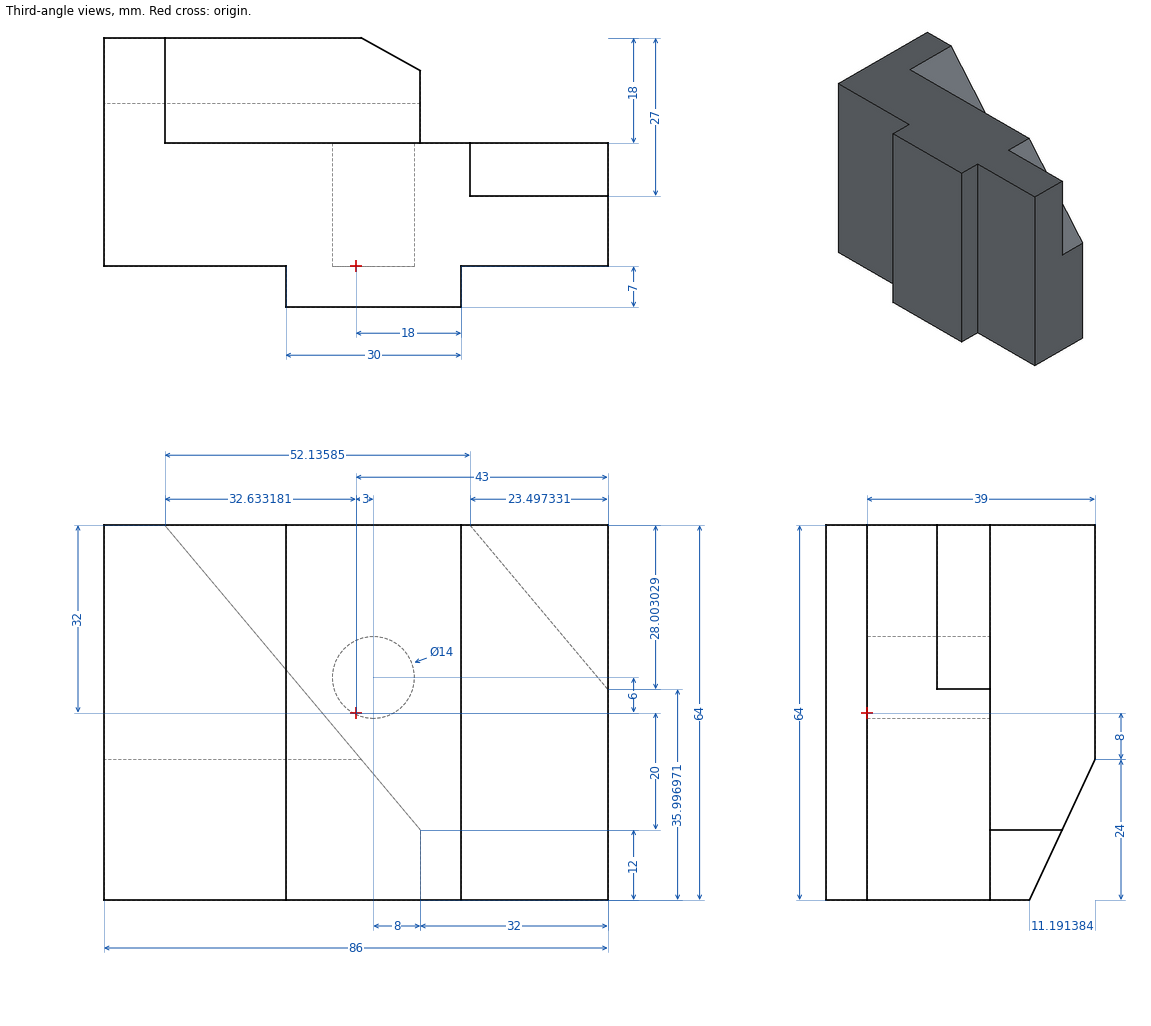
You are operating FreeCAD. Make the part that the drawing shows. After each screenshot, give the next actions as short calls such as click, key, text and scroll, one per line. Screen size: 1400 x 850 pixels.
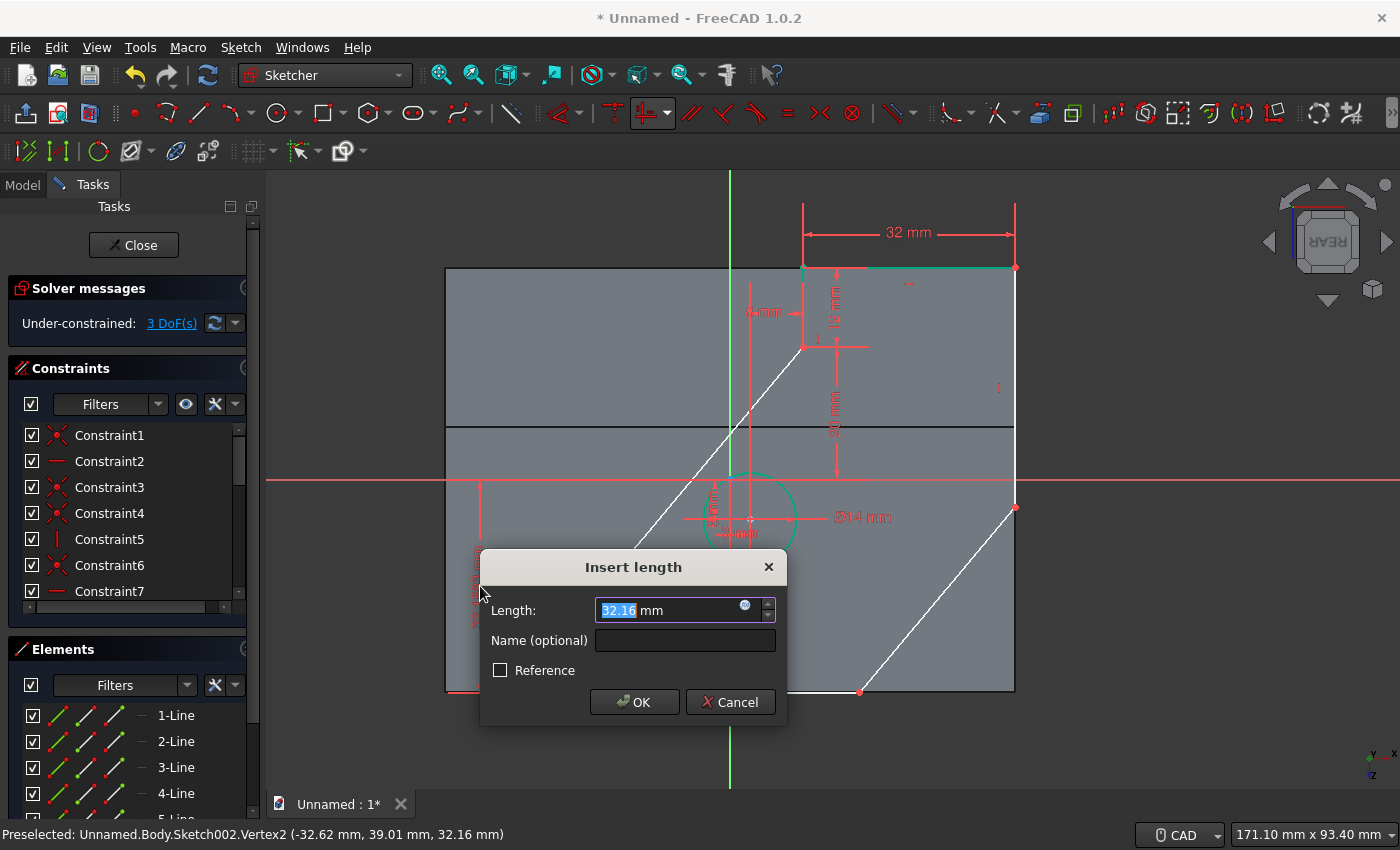
text(32)
key(Return)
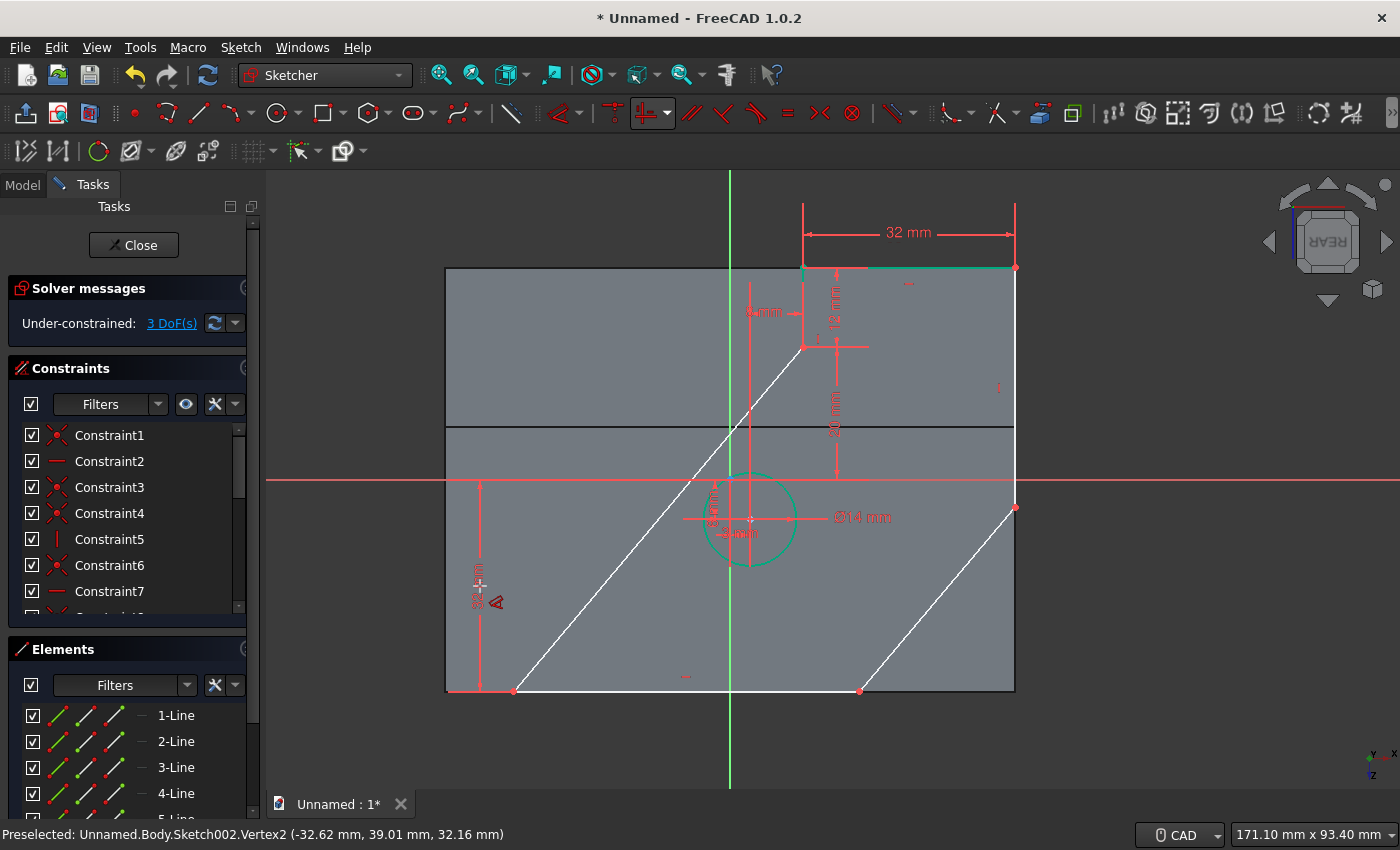
click(618, 692)
click(687, 726)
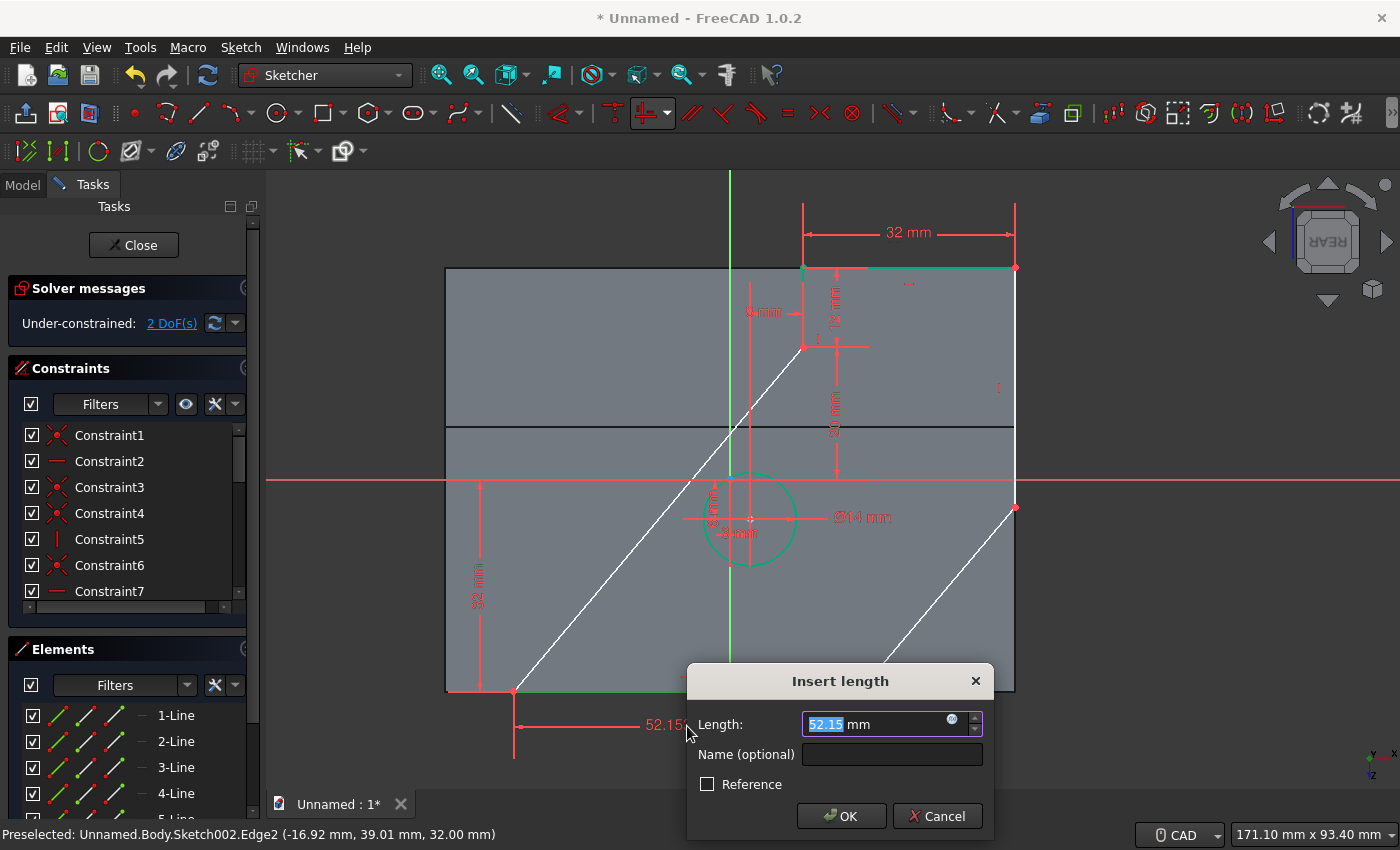
text(52.13585)
key(Return)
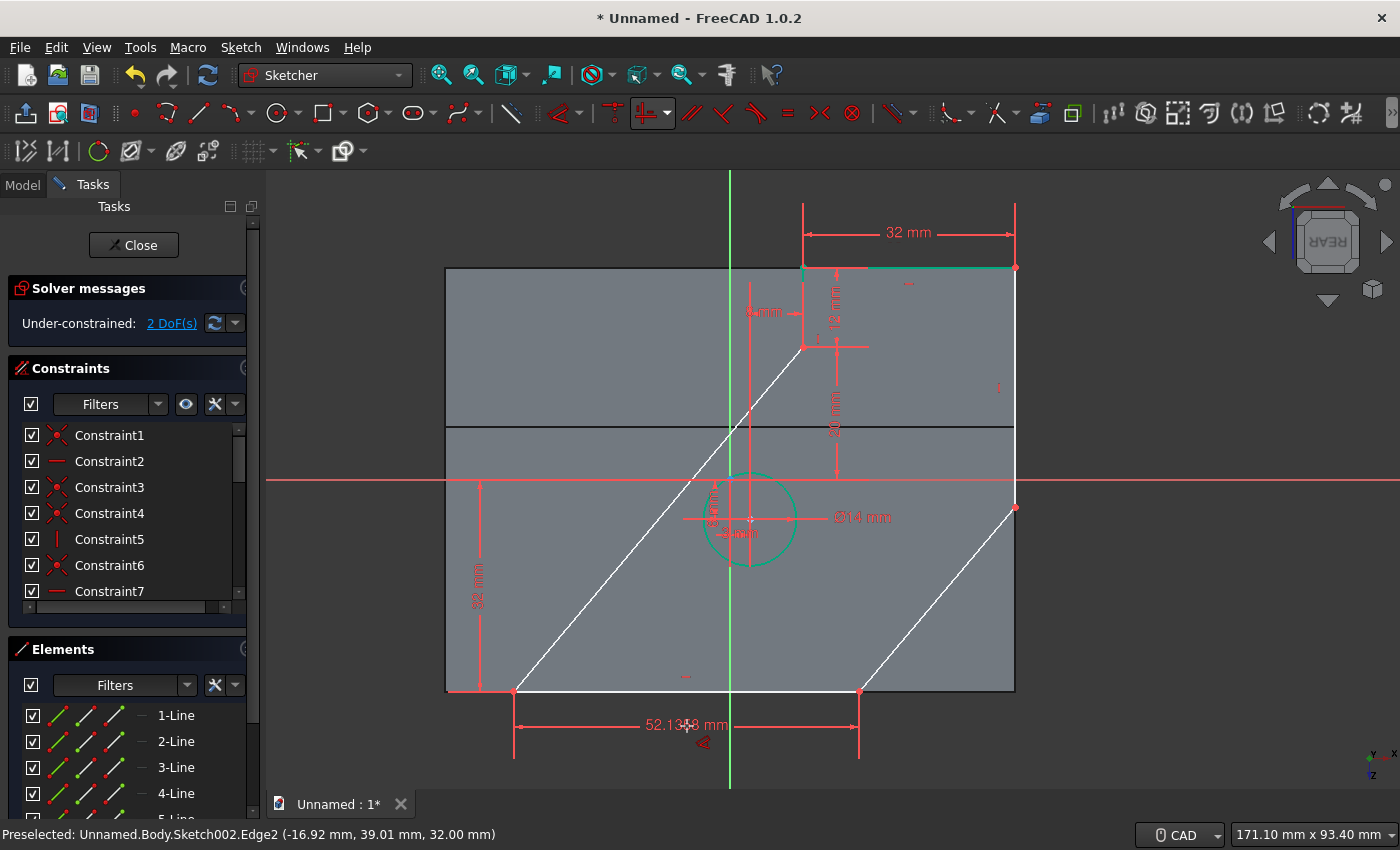
click(1015, 435)
click(1049, 387)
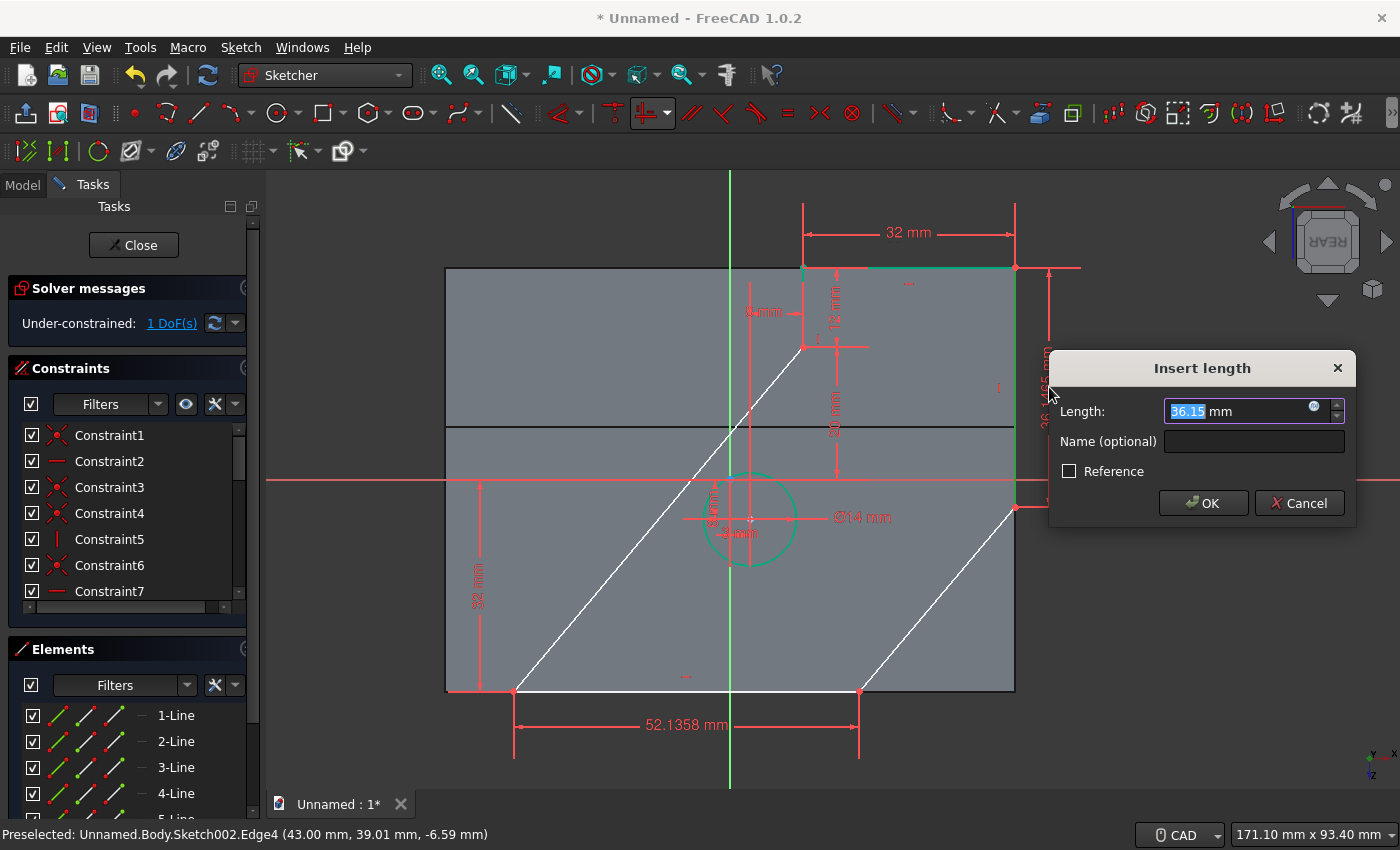
text(35.996971)
key(Return)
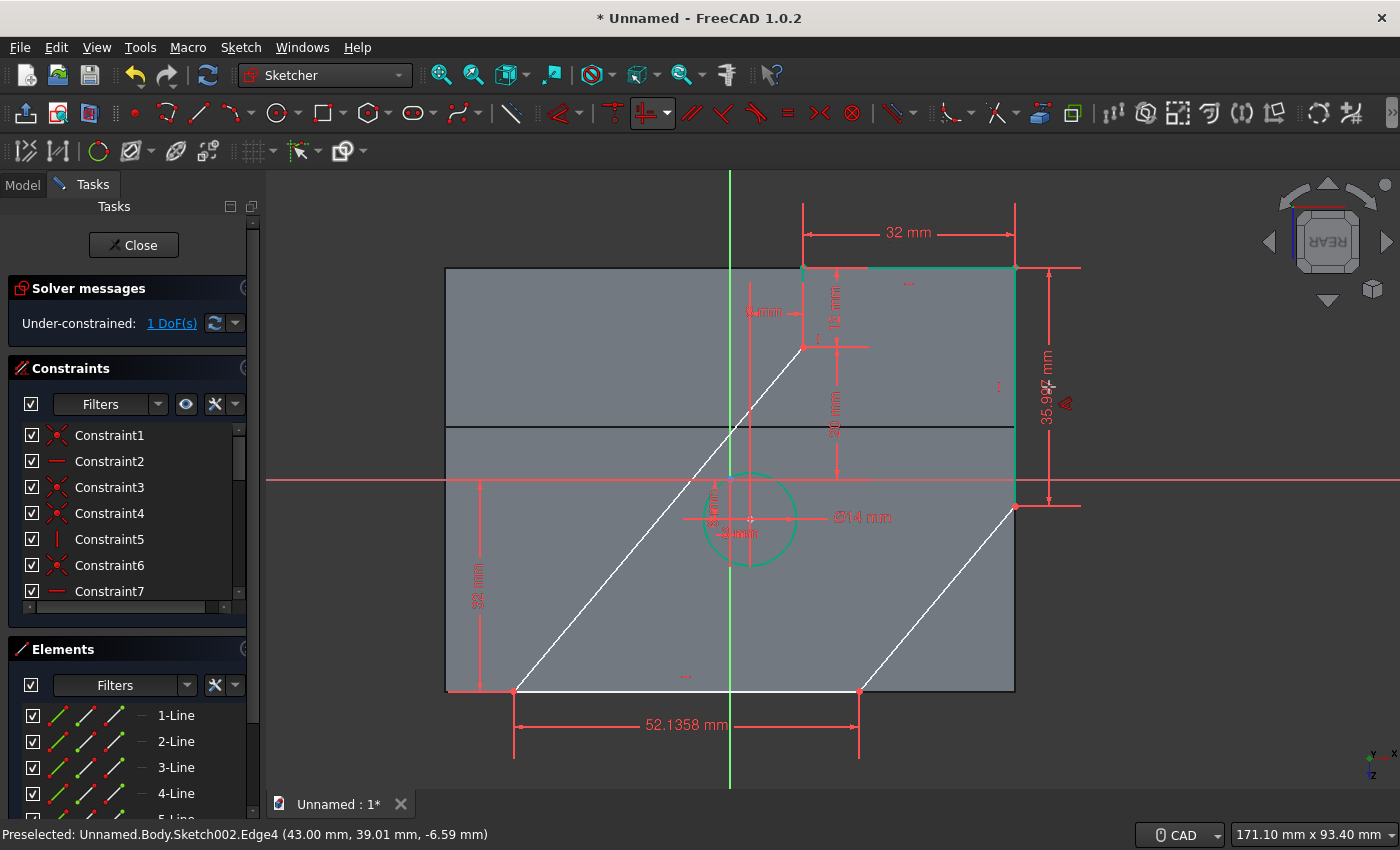
click(514, 692)
click(572, 726)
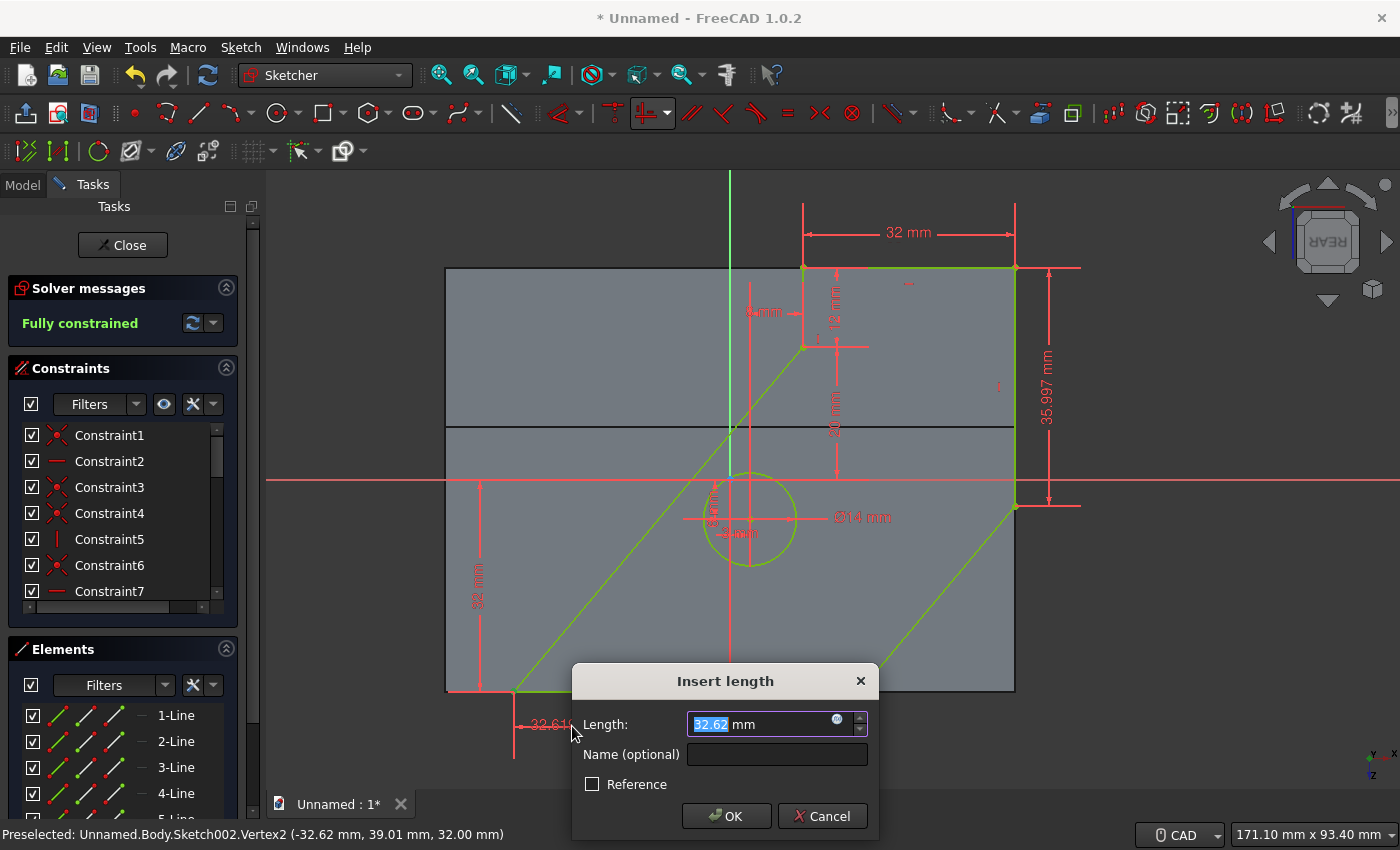
text(32.633181)
key(Return)
key(Escape)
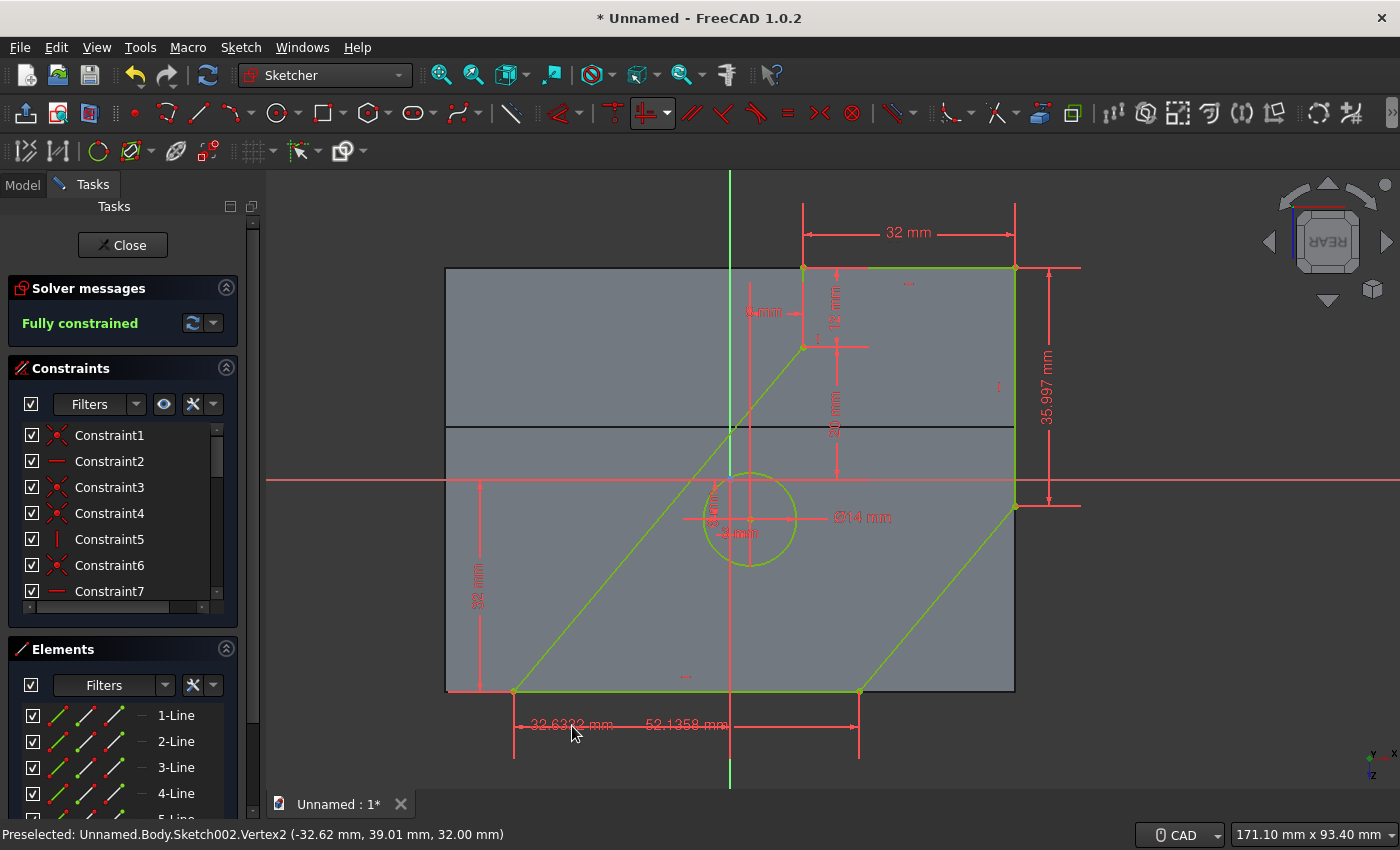
click(123, 245)